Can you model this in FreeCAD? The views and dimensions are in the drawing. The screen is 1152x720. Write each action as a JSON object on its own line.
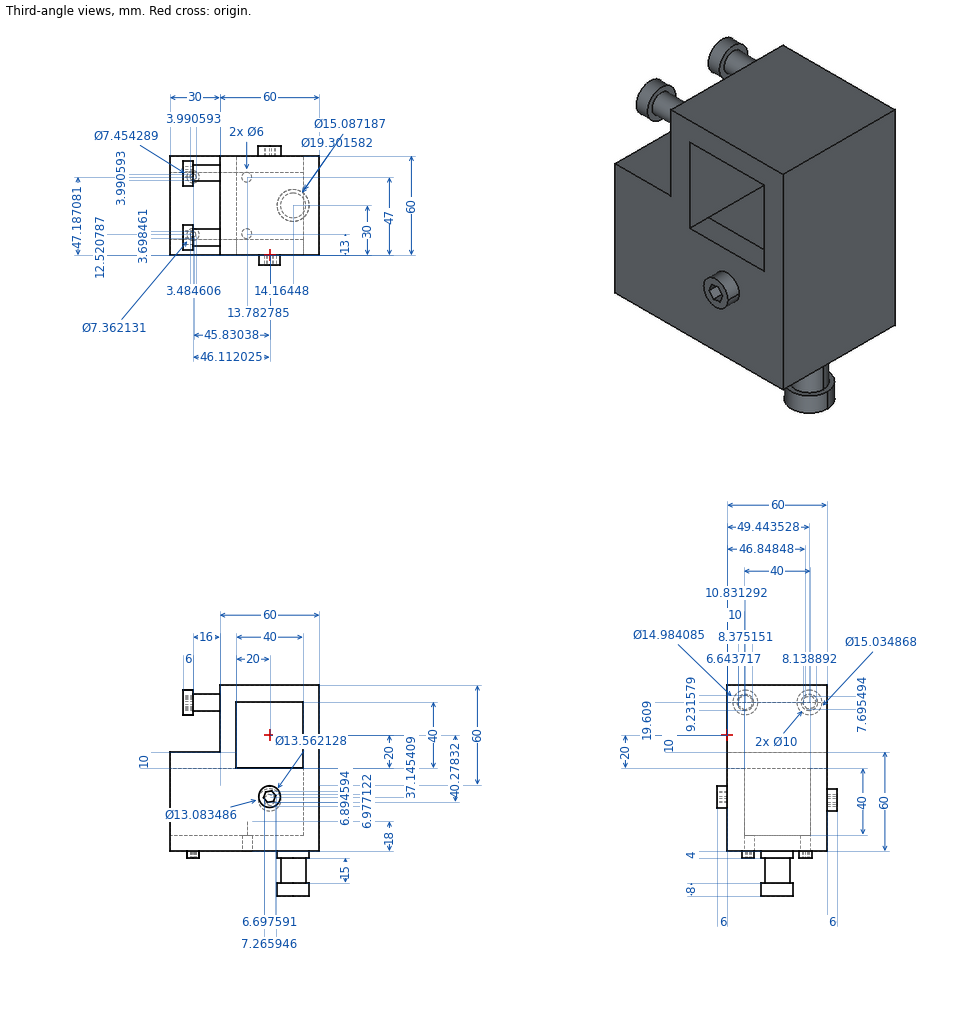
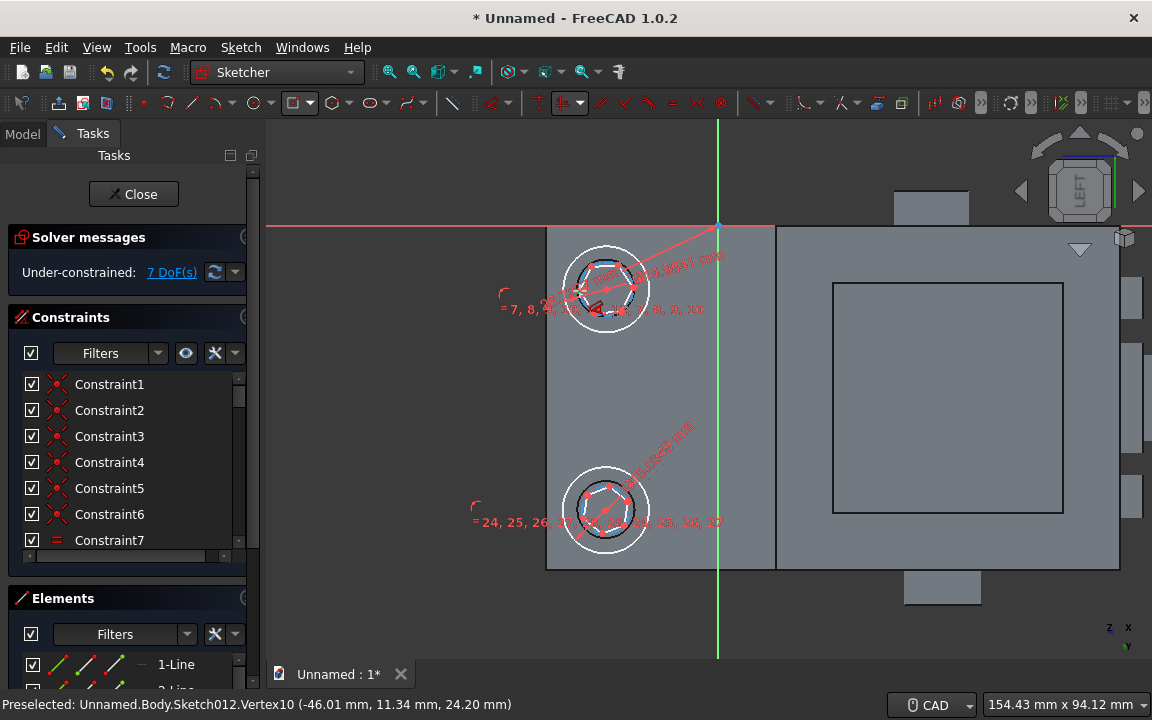
{"action": "left_click", "coordinate": [633, 288]}
{"action": "left_click", "coordinate": [606, 349]}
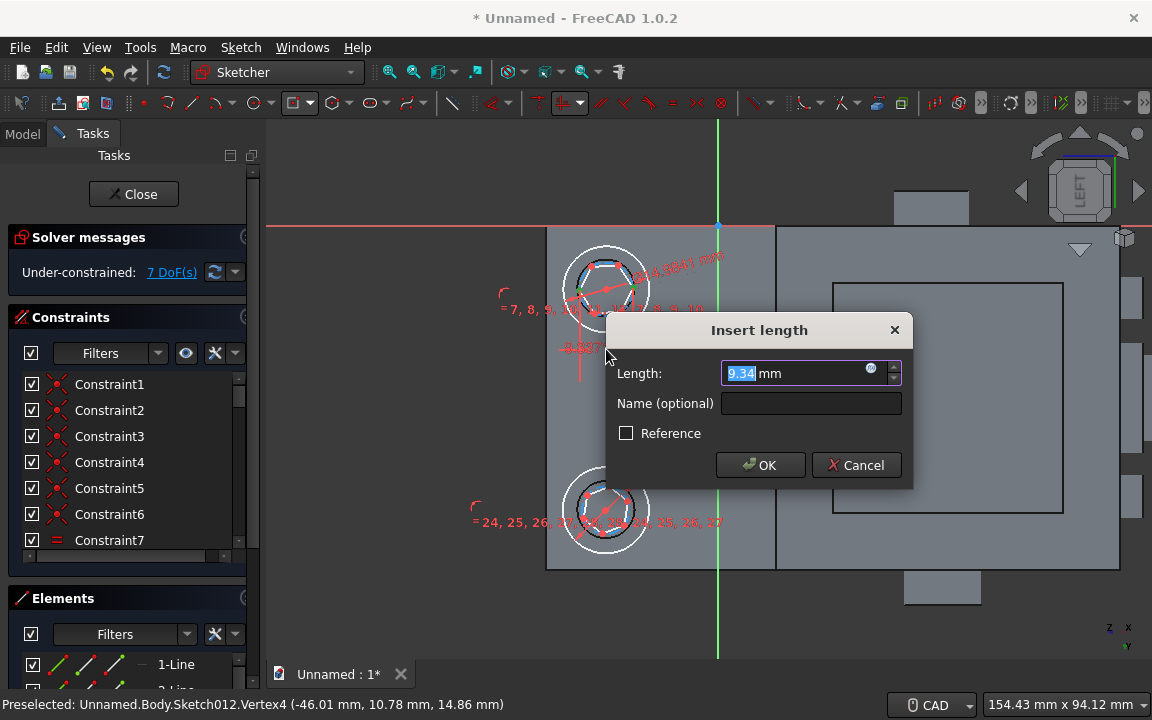
{"action": "type", "text": "9.231579"}
{"action": "key", "text": "Return"}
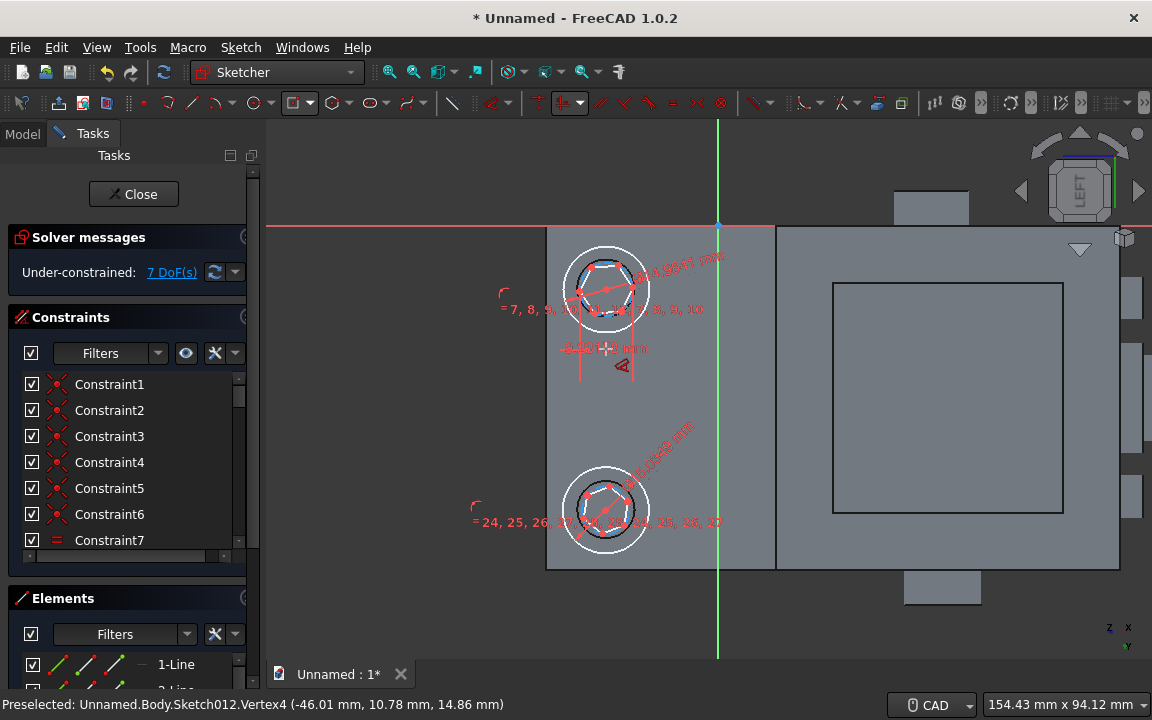
{"action": "left_click", "coordinate": [595, 313]}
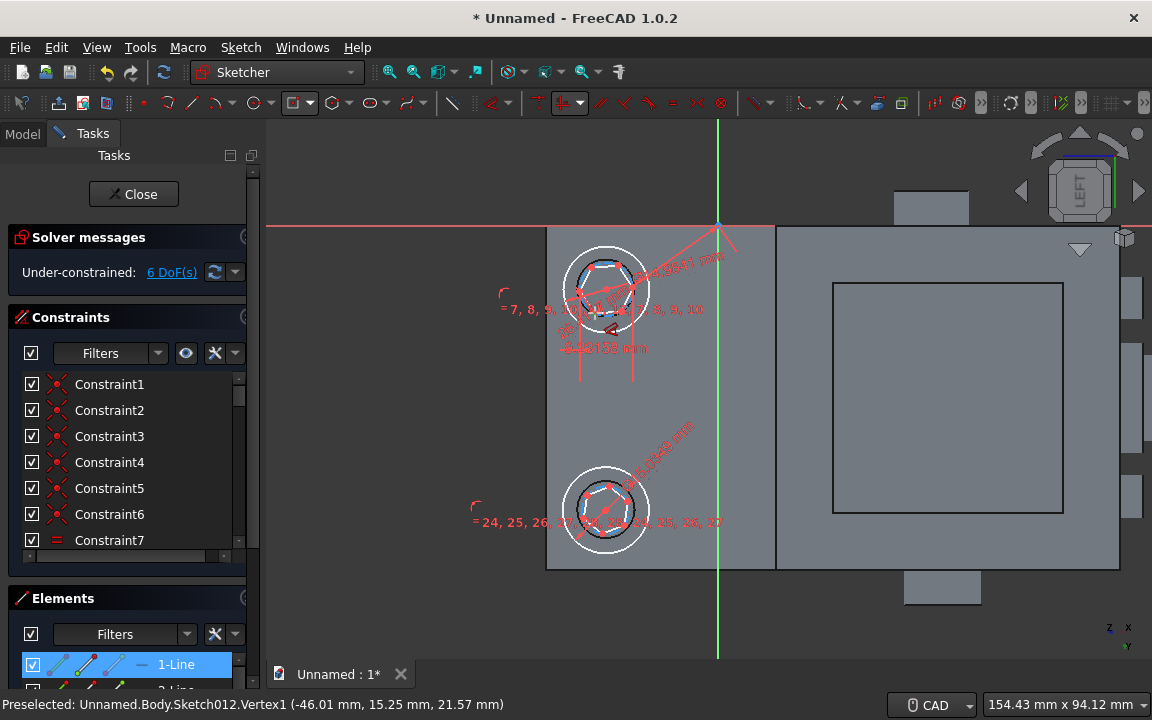
{"action": "left_click", "coordinate": [618, 266]}
{"action": "left_click", "coordinate": [537, 290]}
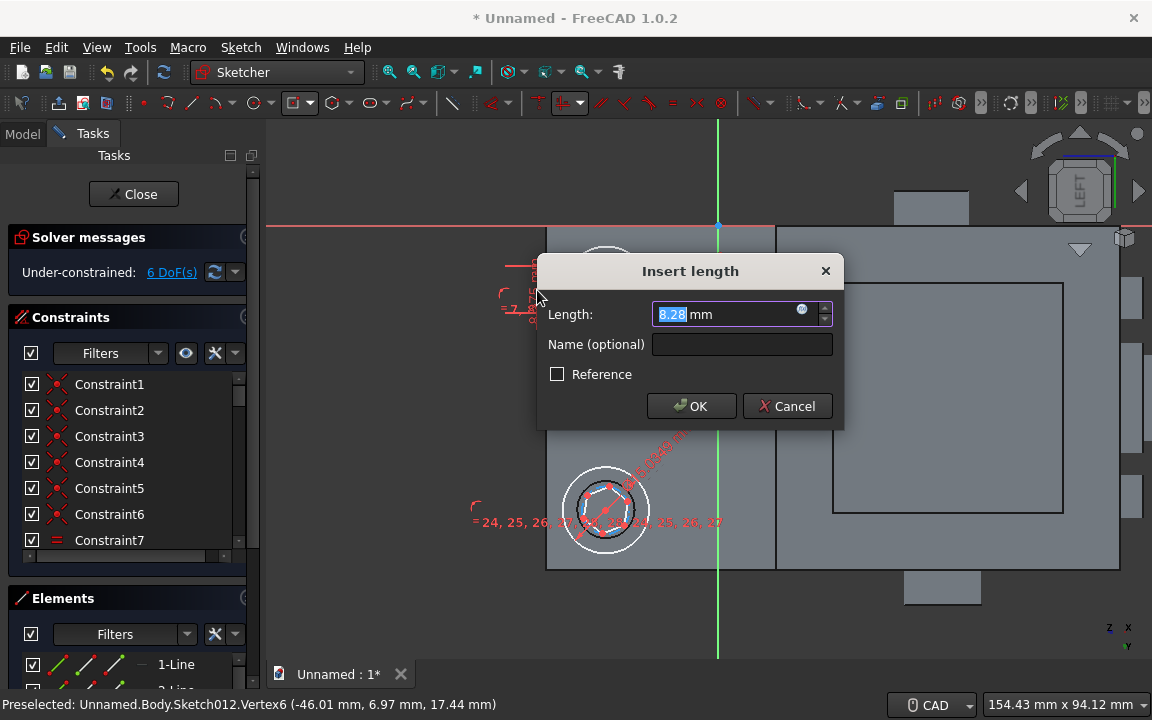
{"action": "type", "text": "8.375151"}
{"action": "key", "text": "Return"}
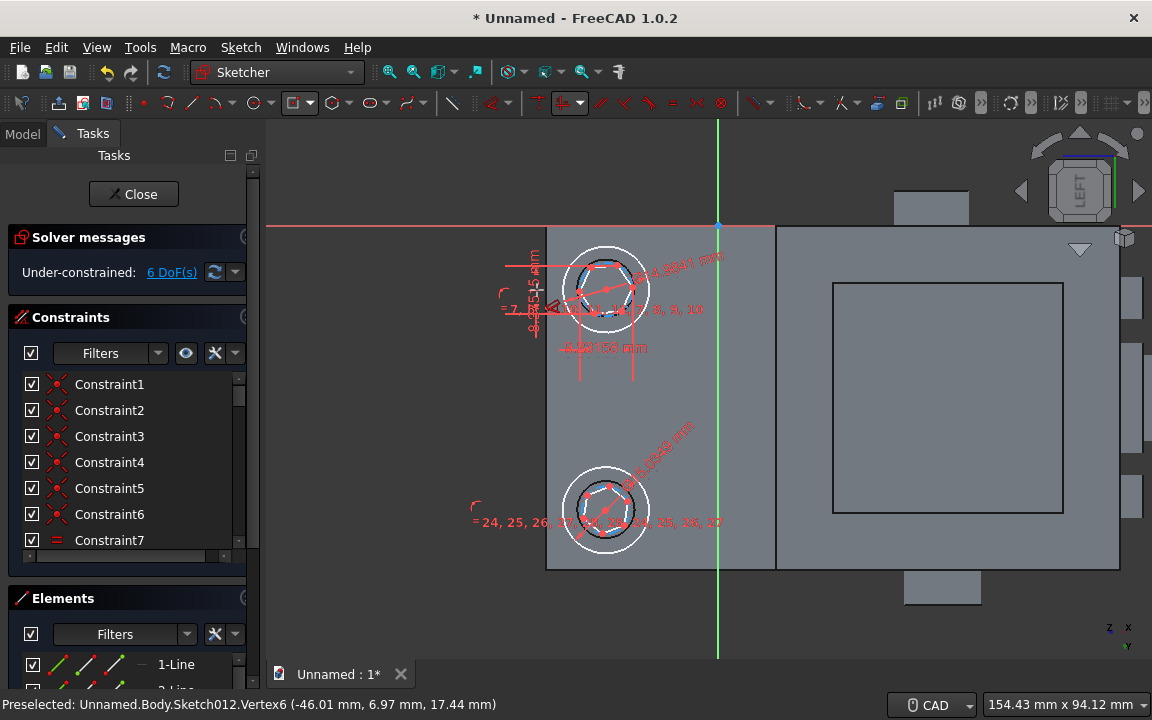
{"action": "left_click", "coordinate": [584, 519]}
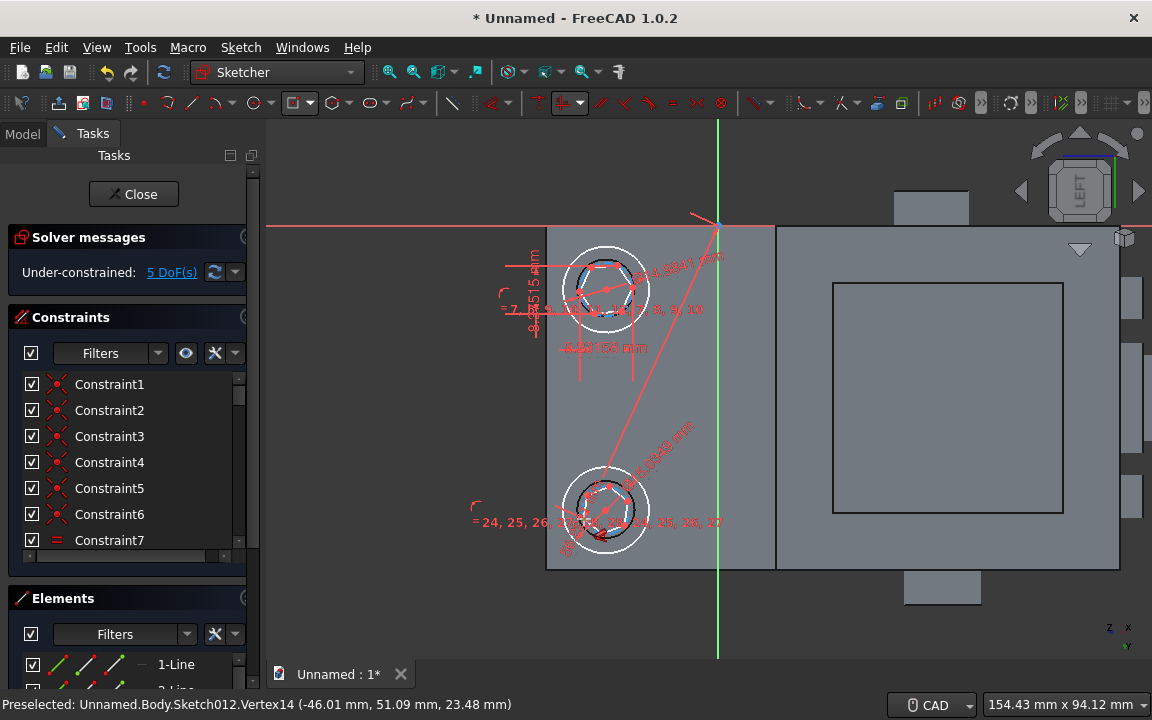
{"action": "left_click", "coordinate": [628, 502]}
{"action": "left_click", "coordinate": [606, 577]}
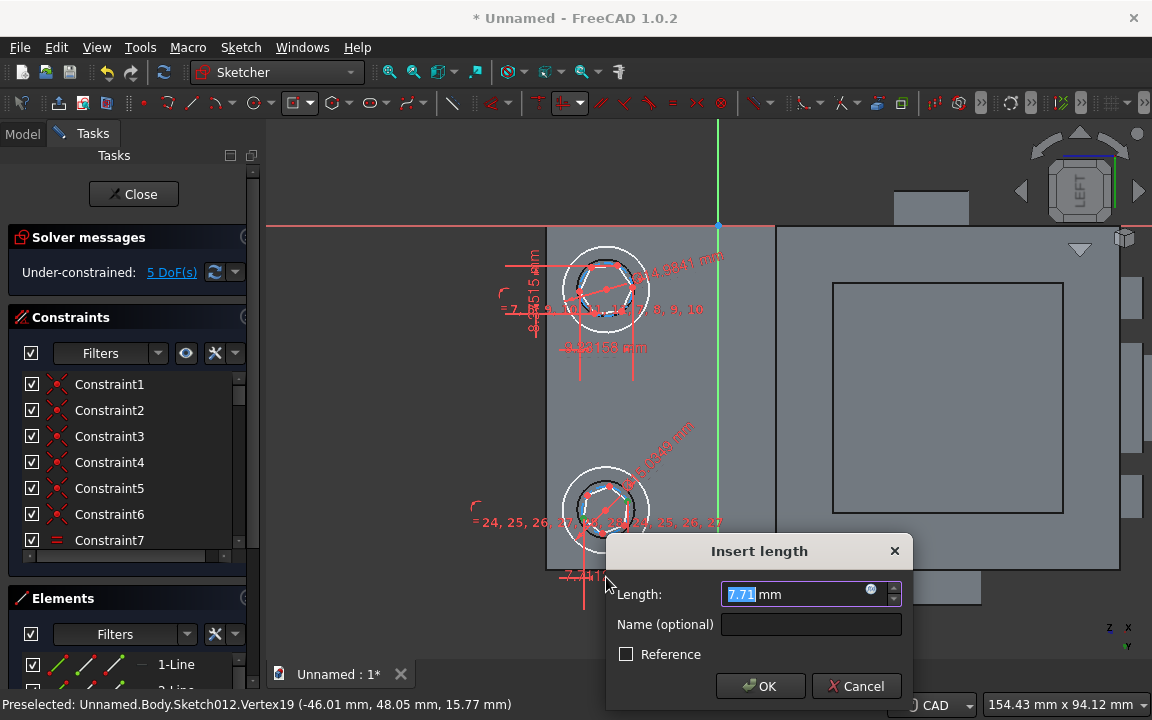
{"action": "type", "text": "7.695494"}
{"action": "key", "text": "Return"}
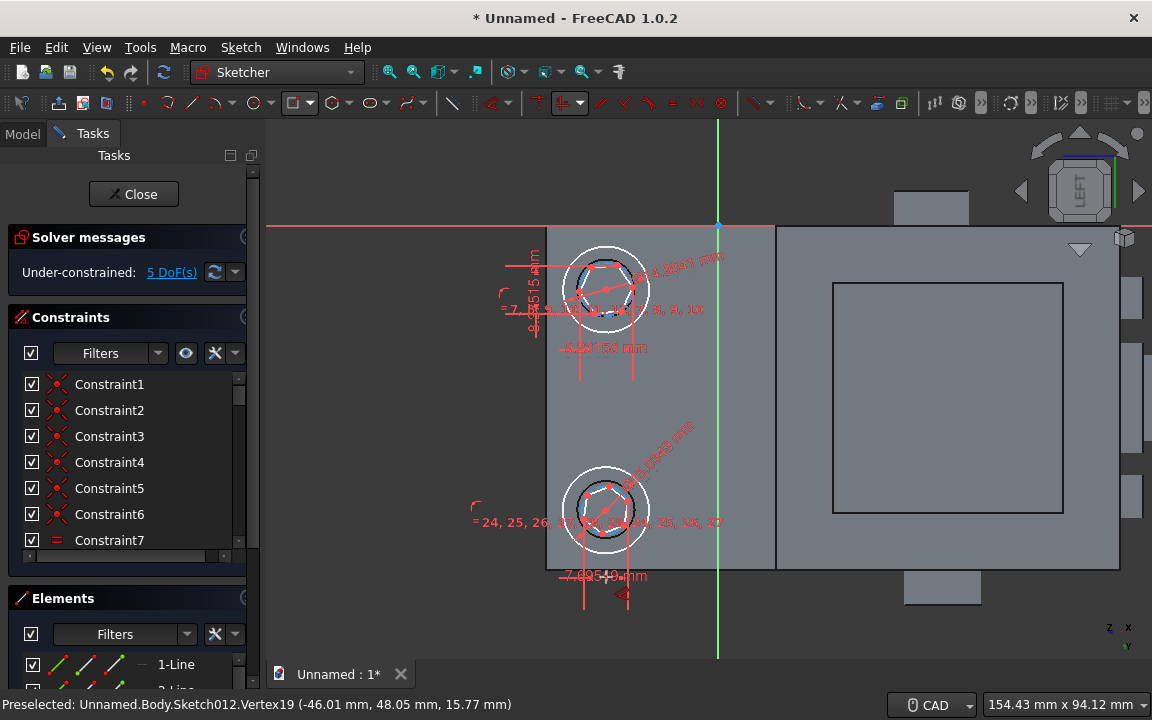
{"action": "left_click", "coordinate": [602, 534]}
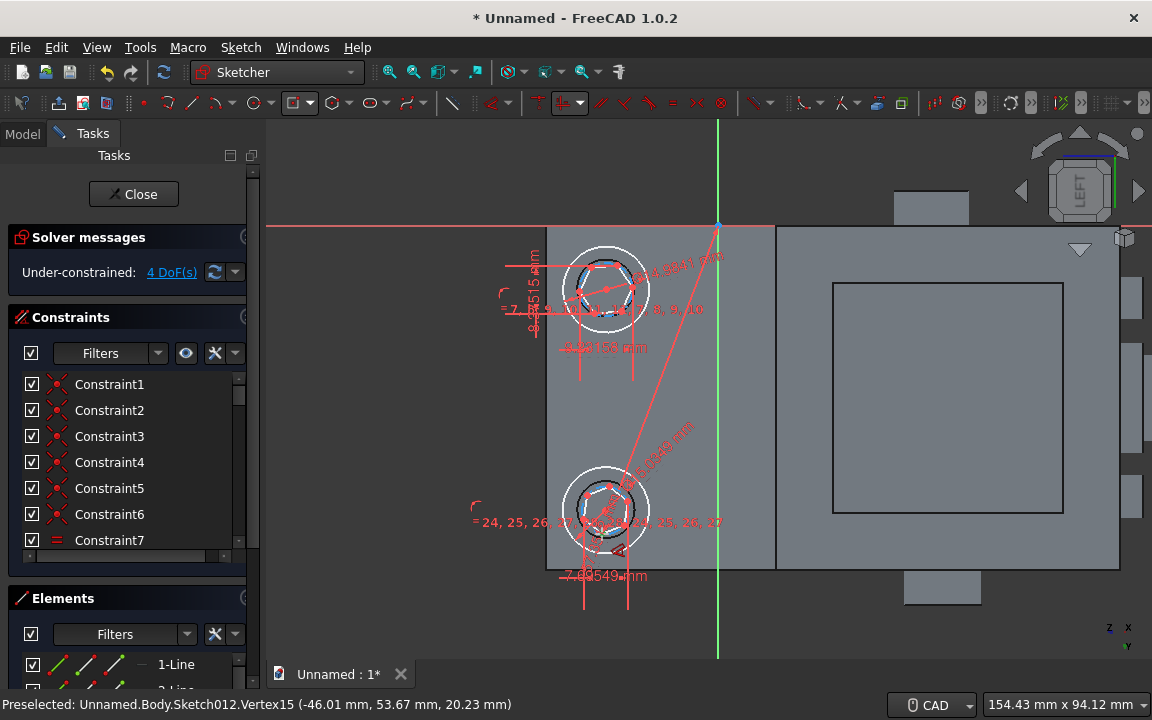
{"action": "left_click", "coordinate": [609, 487]}
{"action": "left_click", "coordinate": [544, 510]}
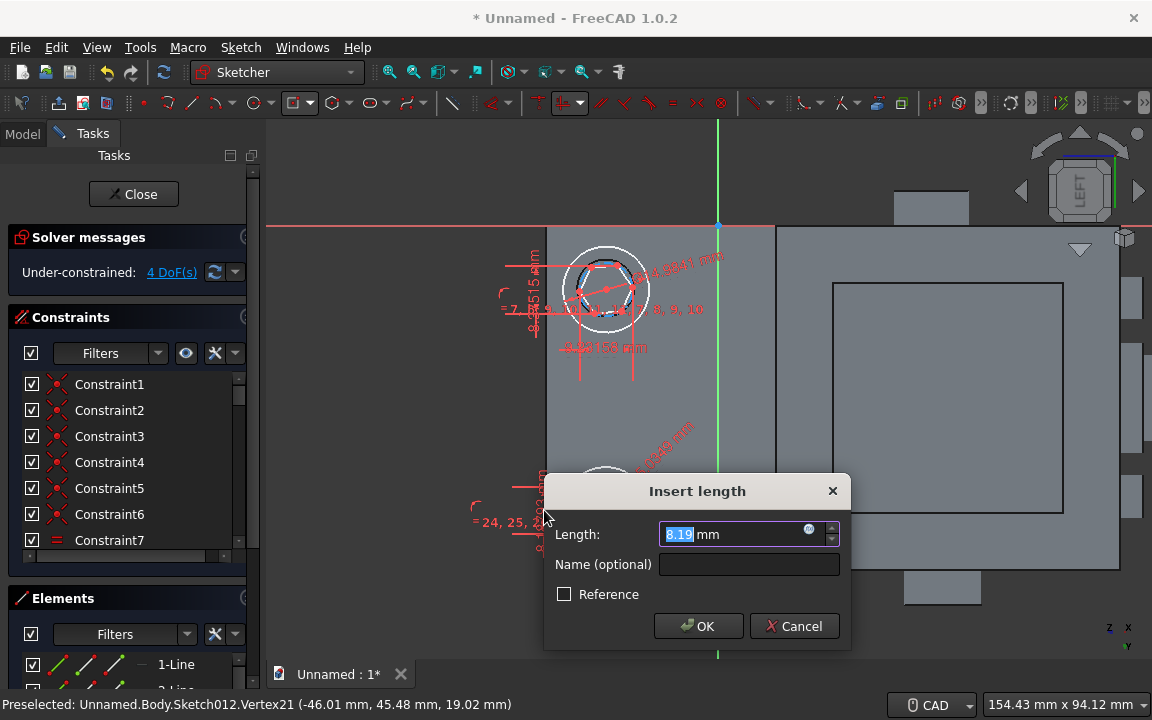
{"action": "type", "text": "8.138892"}
{"action": "key", "text": "Return"}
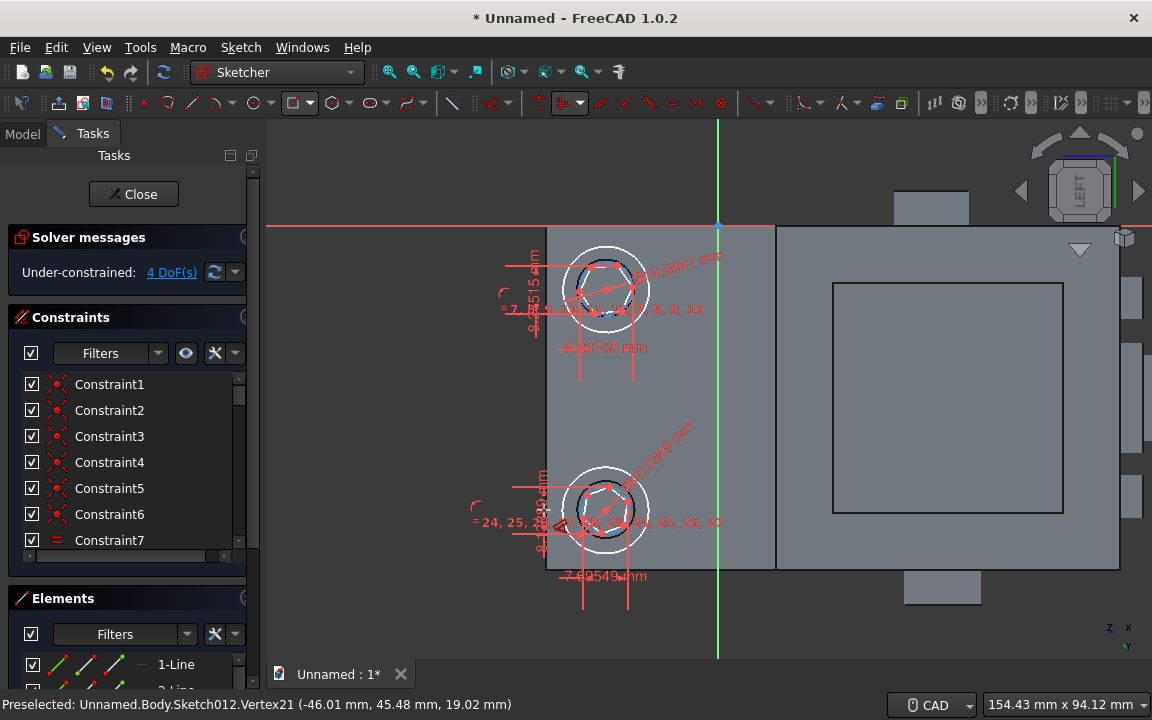
{"action": "left_click", "coordinate": [606, 290]}
{"action": "left_click", "coordinate": [662, 192]}